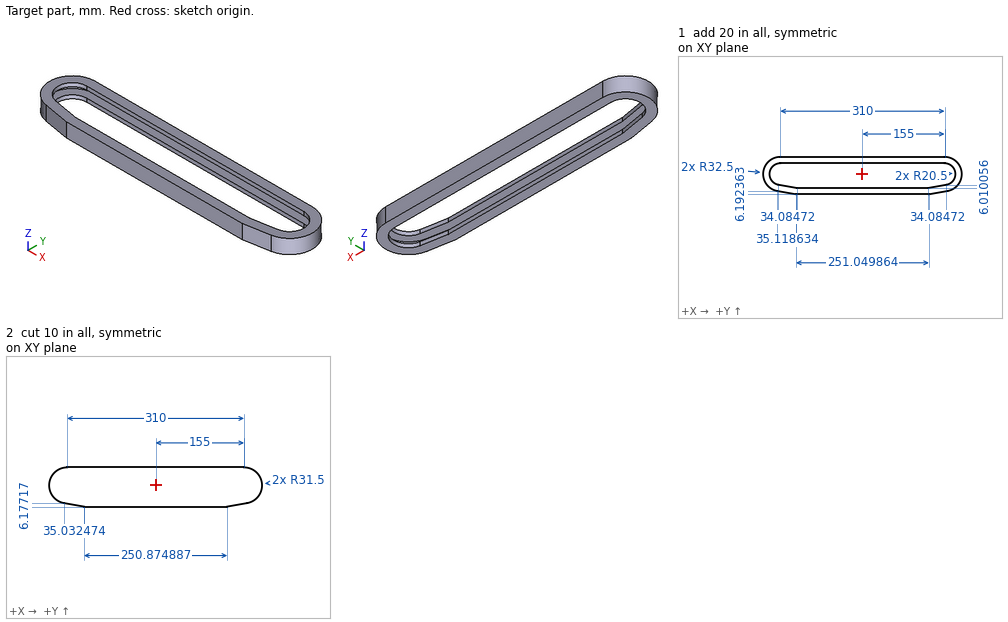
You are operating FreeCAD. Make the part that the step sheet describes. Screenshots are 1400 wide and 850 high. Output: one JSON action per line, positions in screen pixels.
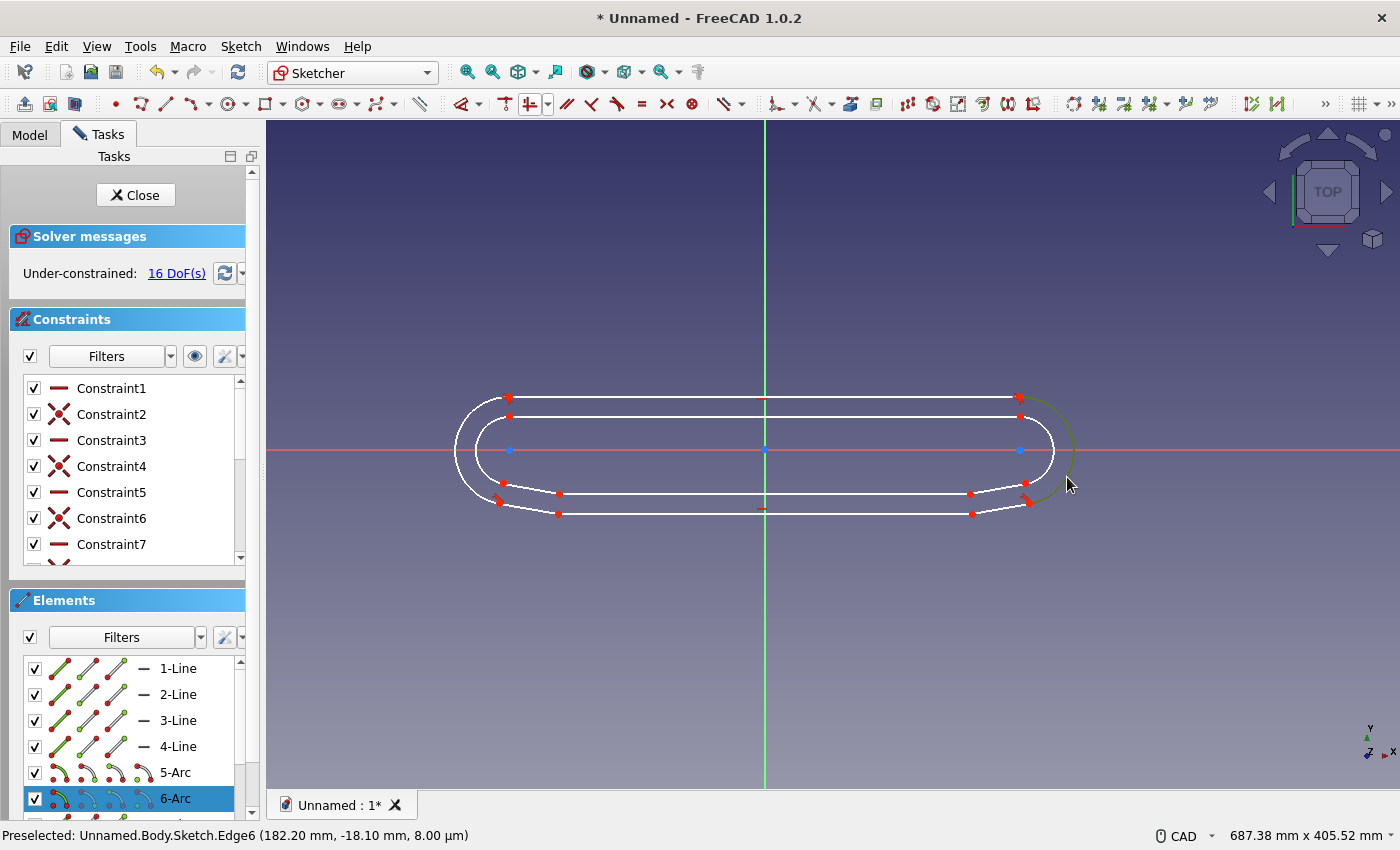
{"action": "left_click", "coordinate": [1050, 467]}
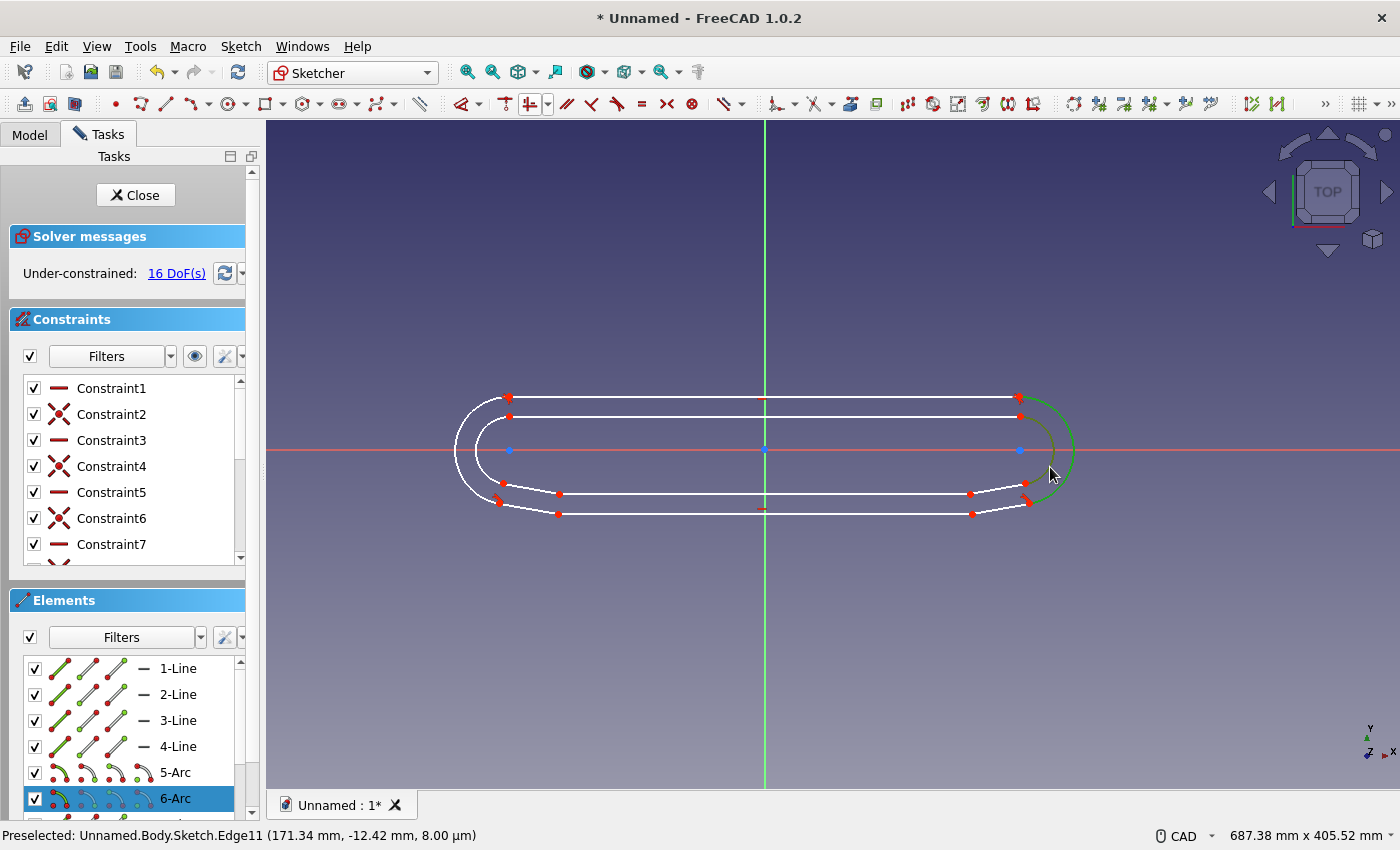
{"action": "key", "text": "c"}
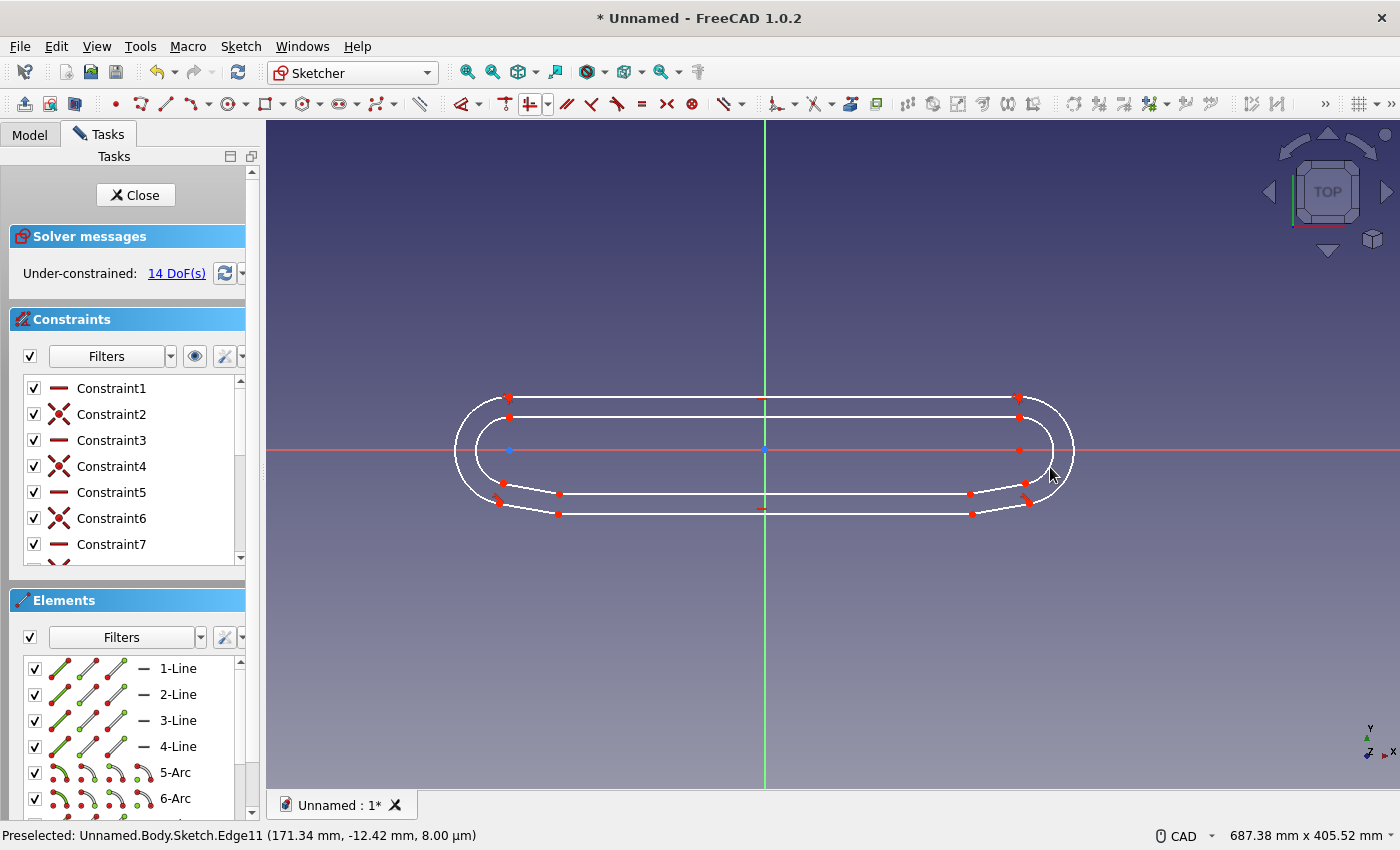
{"action": "left_click", "coordinate": [467, 417]}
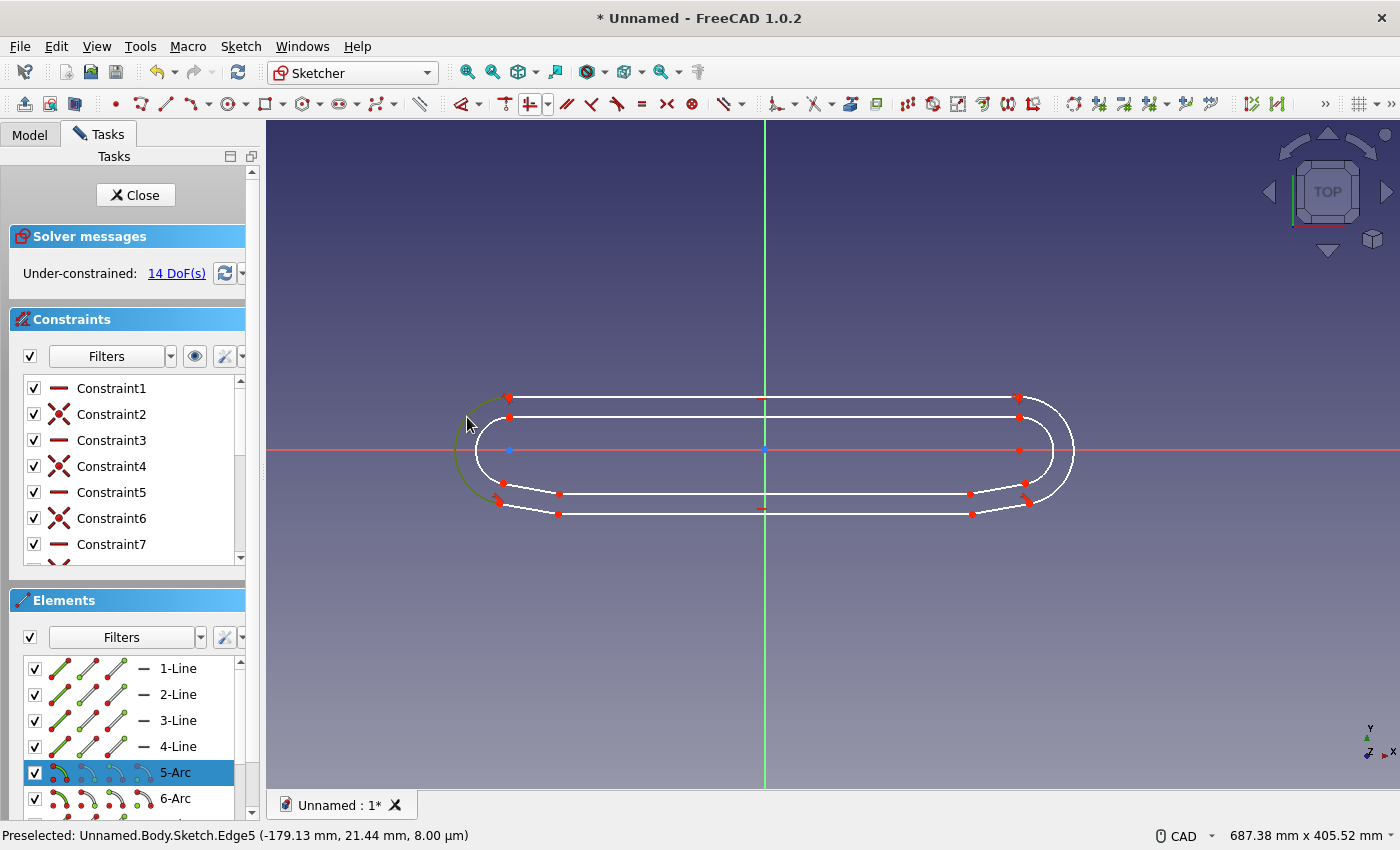
{"action": "left_click", "coordinate": [484, 430]}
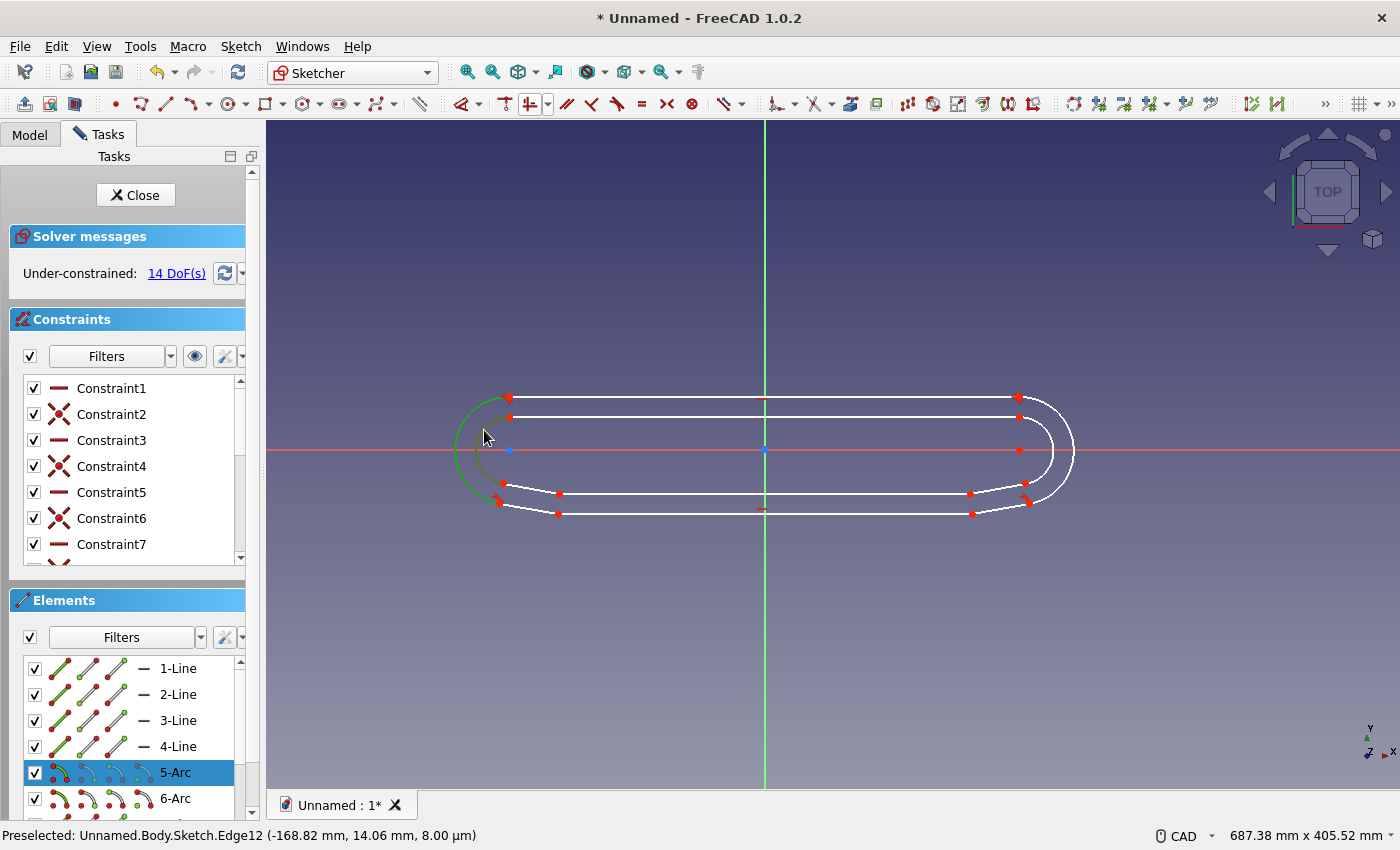
{"action": "key", "text": "c"}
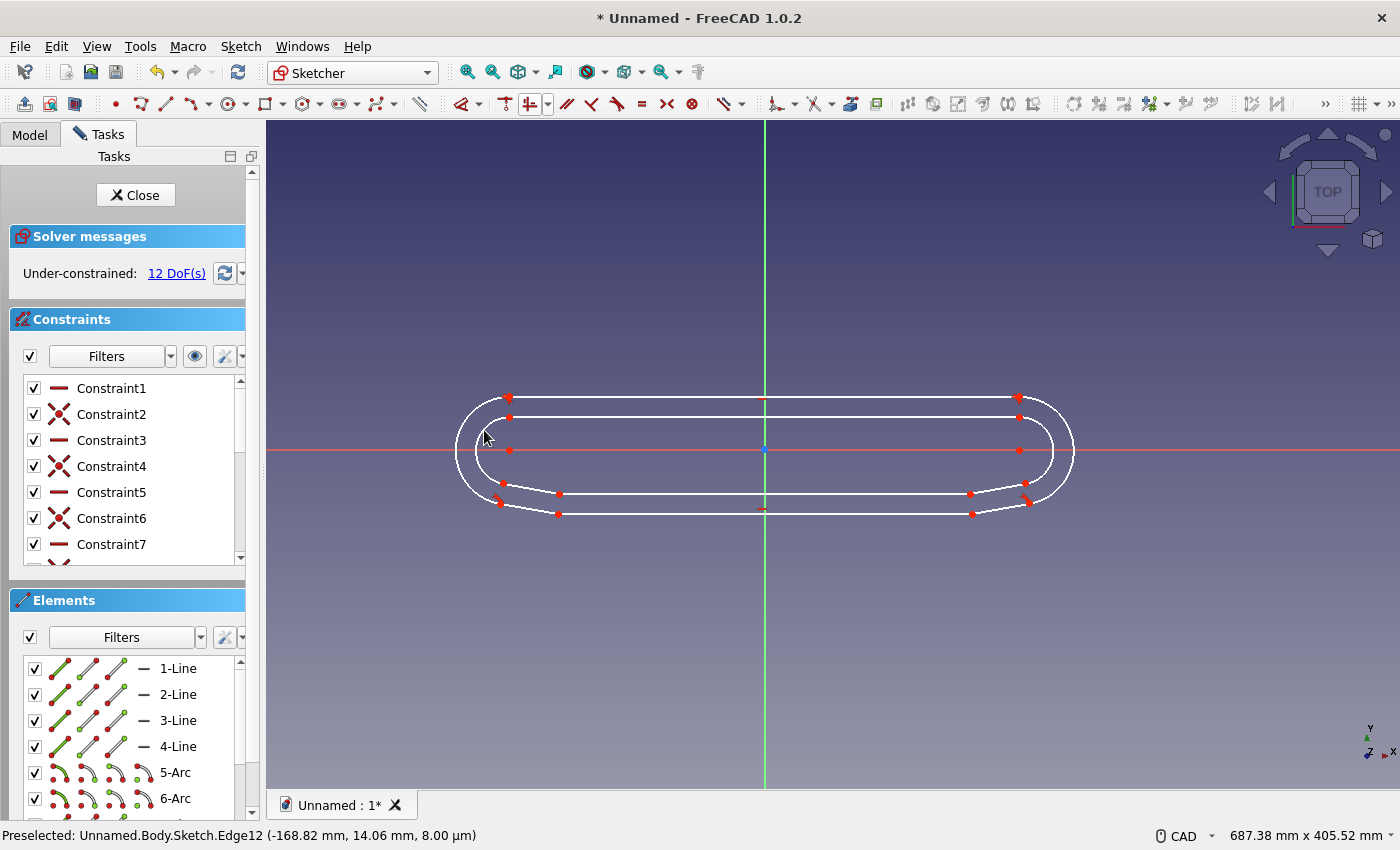
{"action": "left_click", "coordinate": [468, 417]}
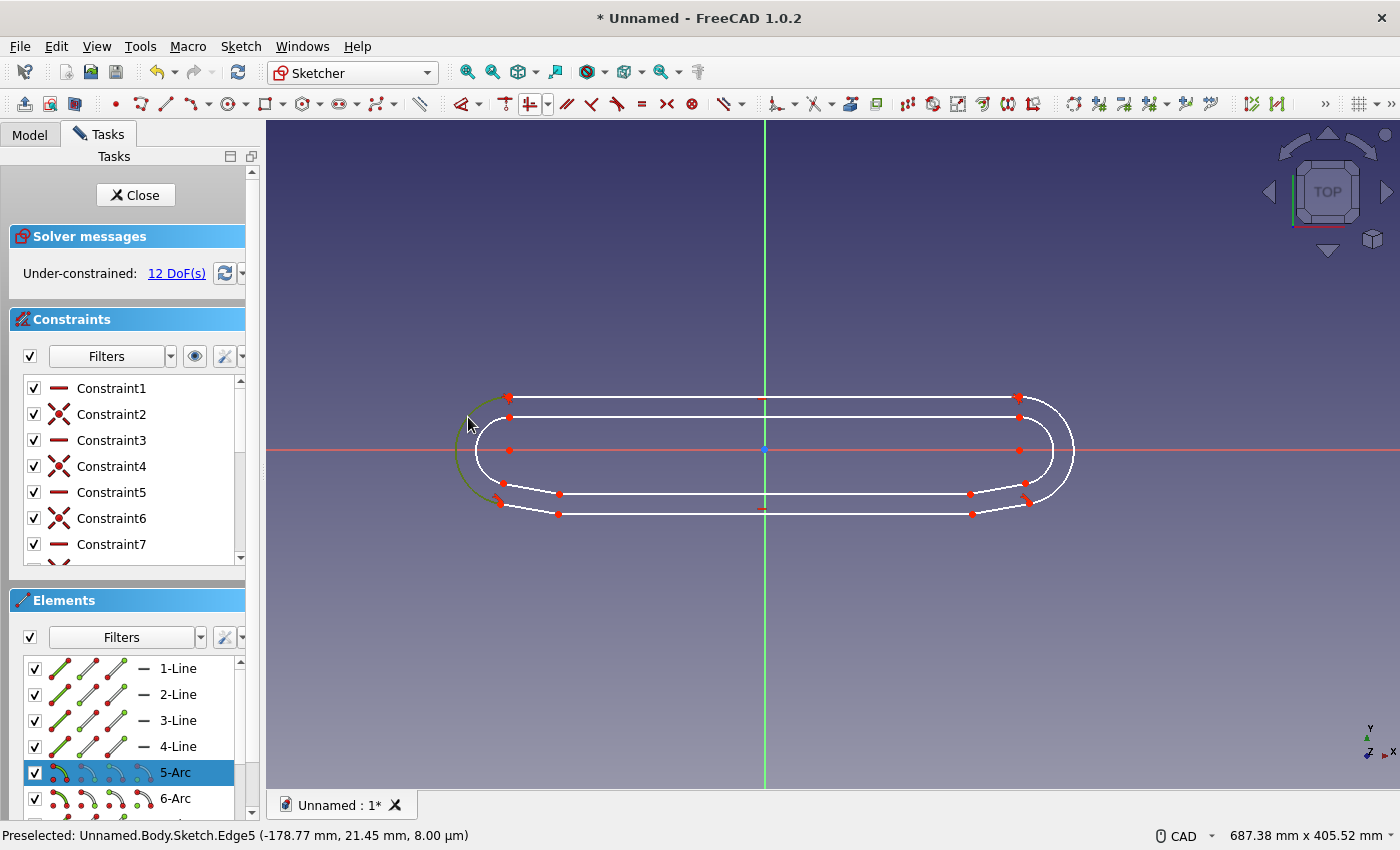
{"action": "left_click", "coordinate": [1067, 477]}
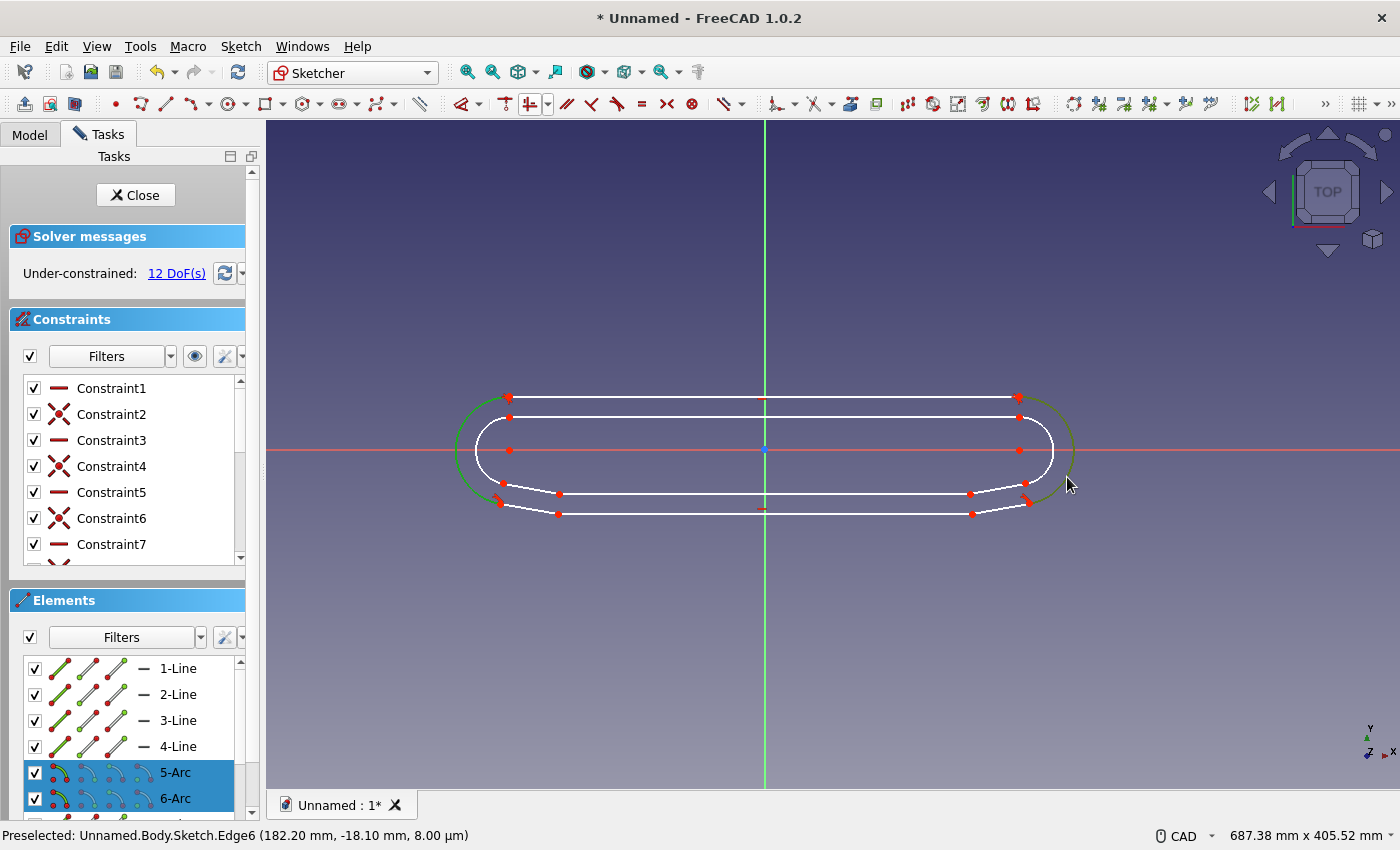
{"action": "left_click", "coordinate": [642, 104]}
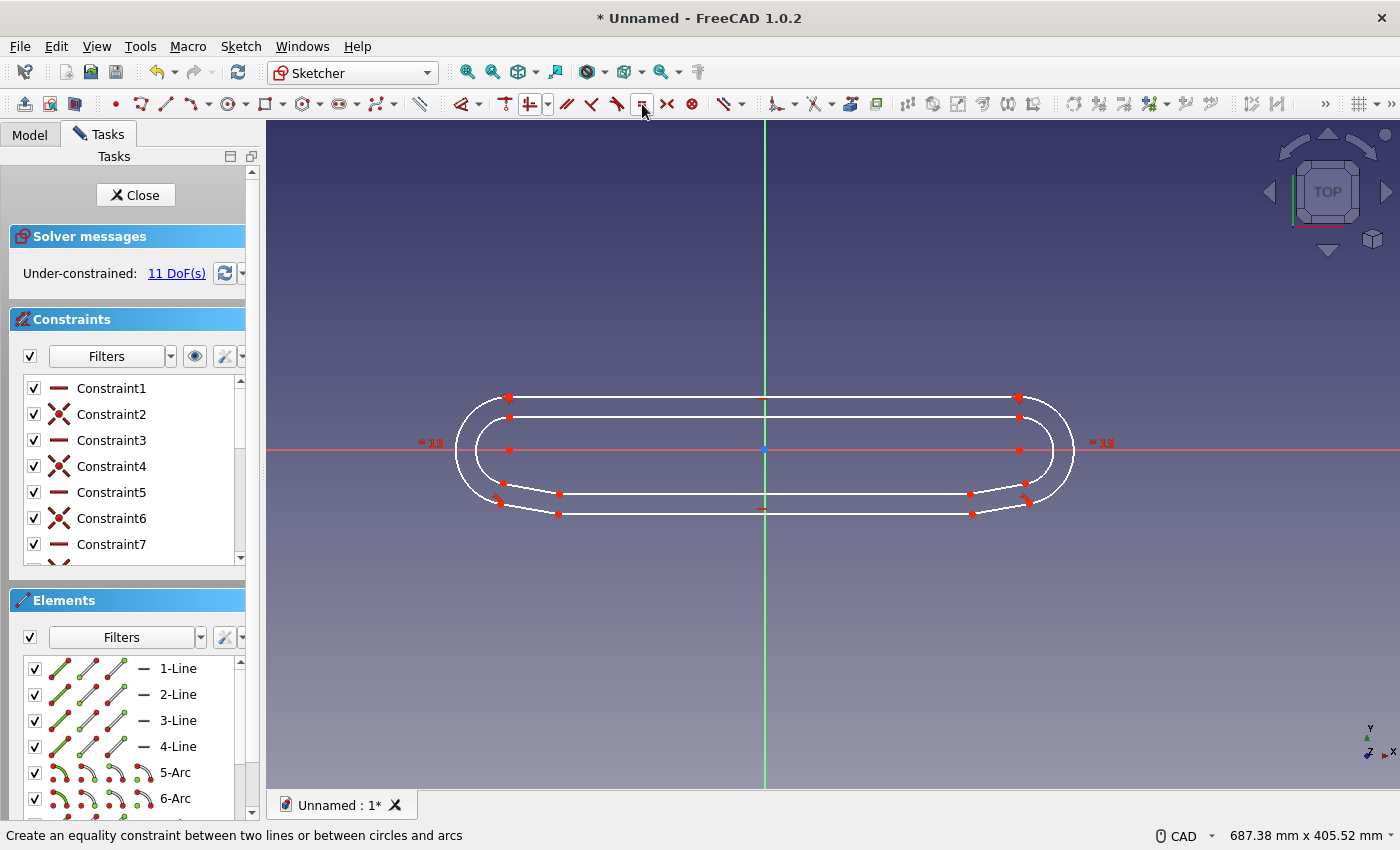
{"action": "left_click", "coordinate": [510, 451]}